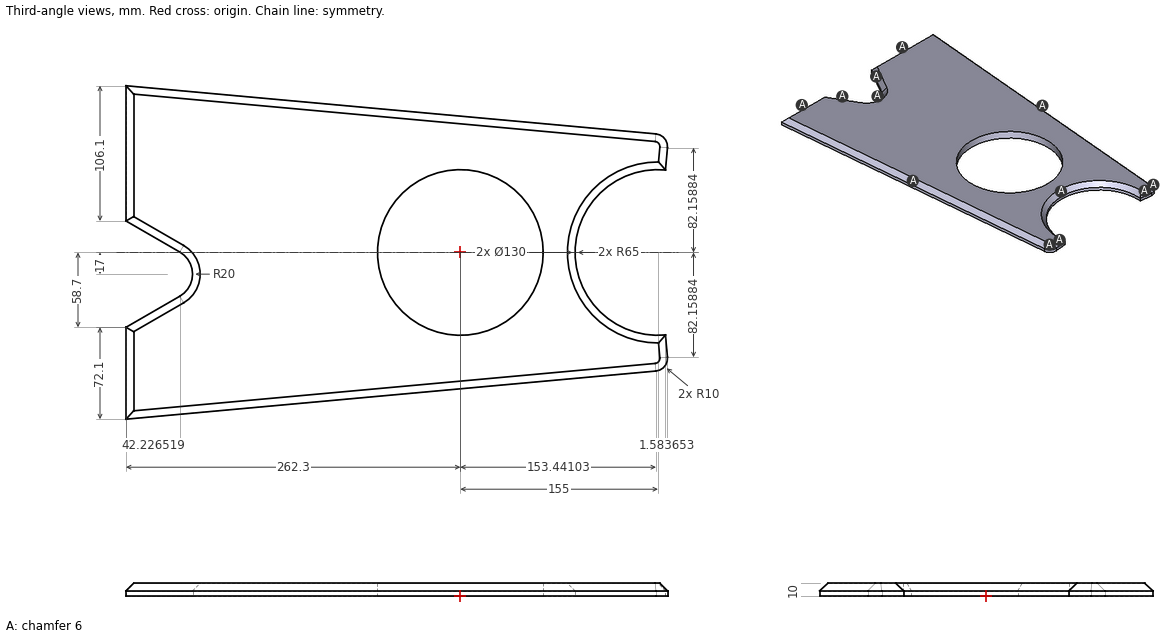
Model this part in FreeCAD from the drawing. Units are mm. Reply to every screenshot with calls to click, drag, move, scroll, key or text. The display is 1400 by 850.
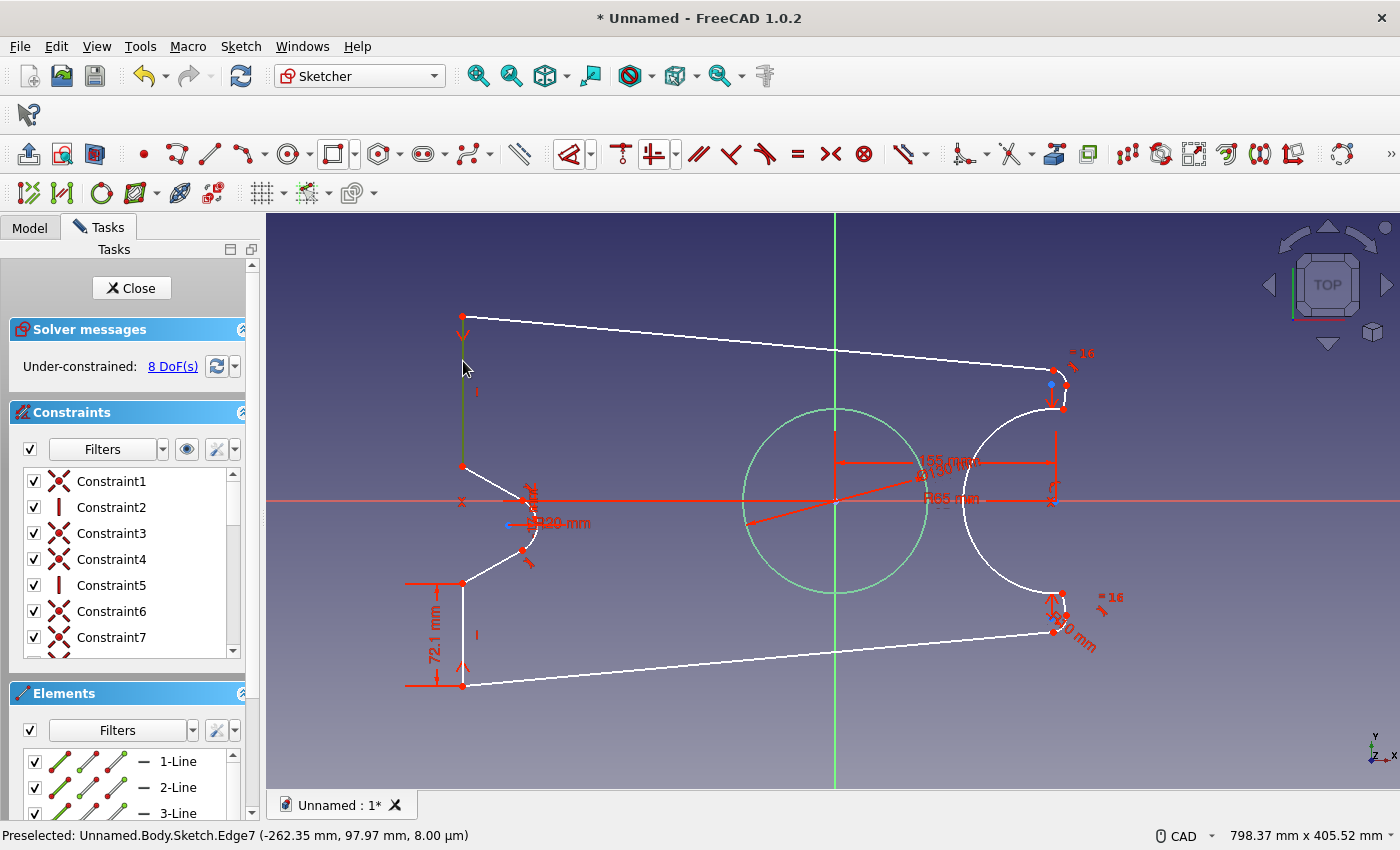
click(590, 154)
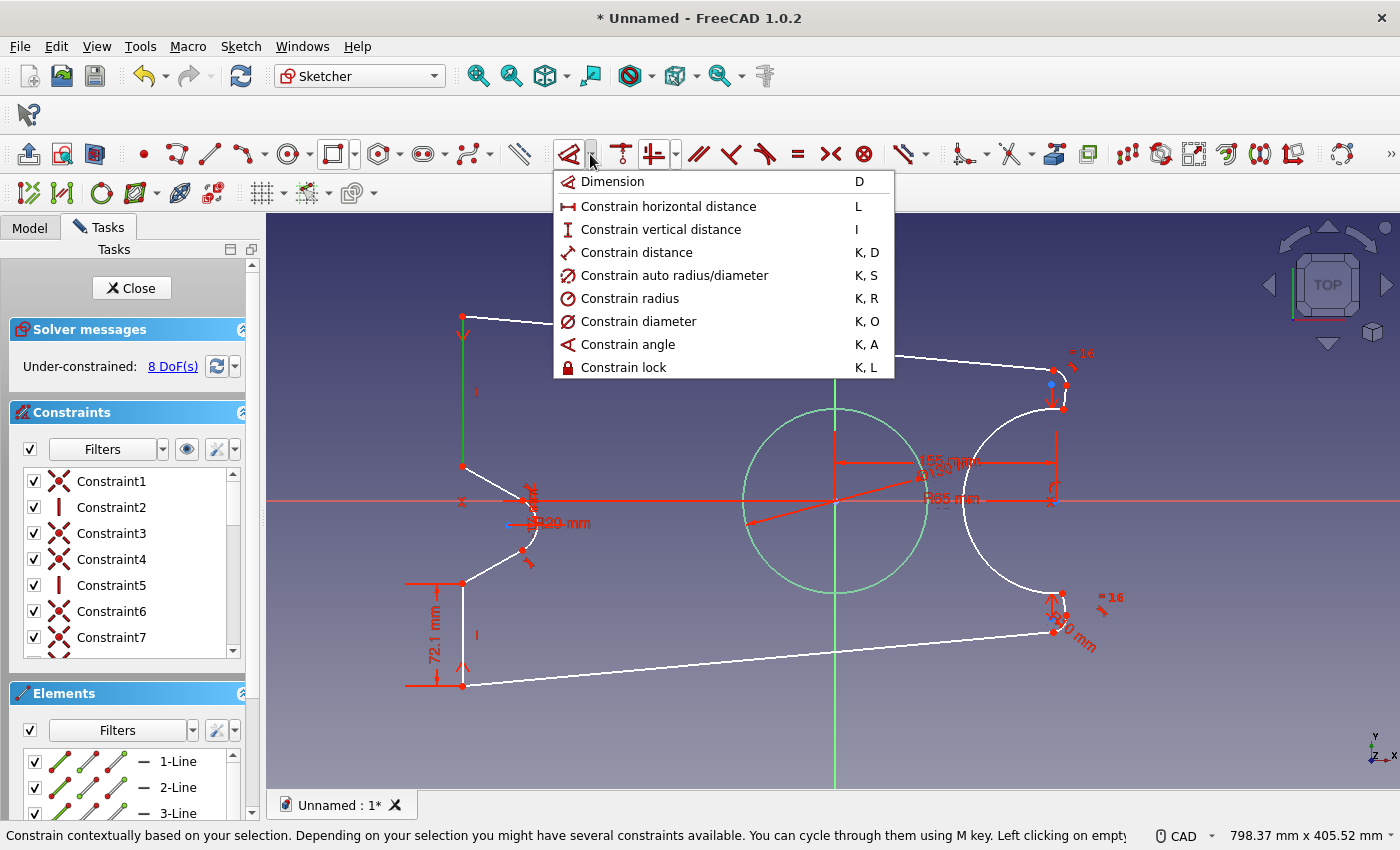
click(724, 230)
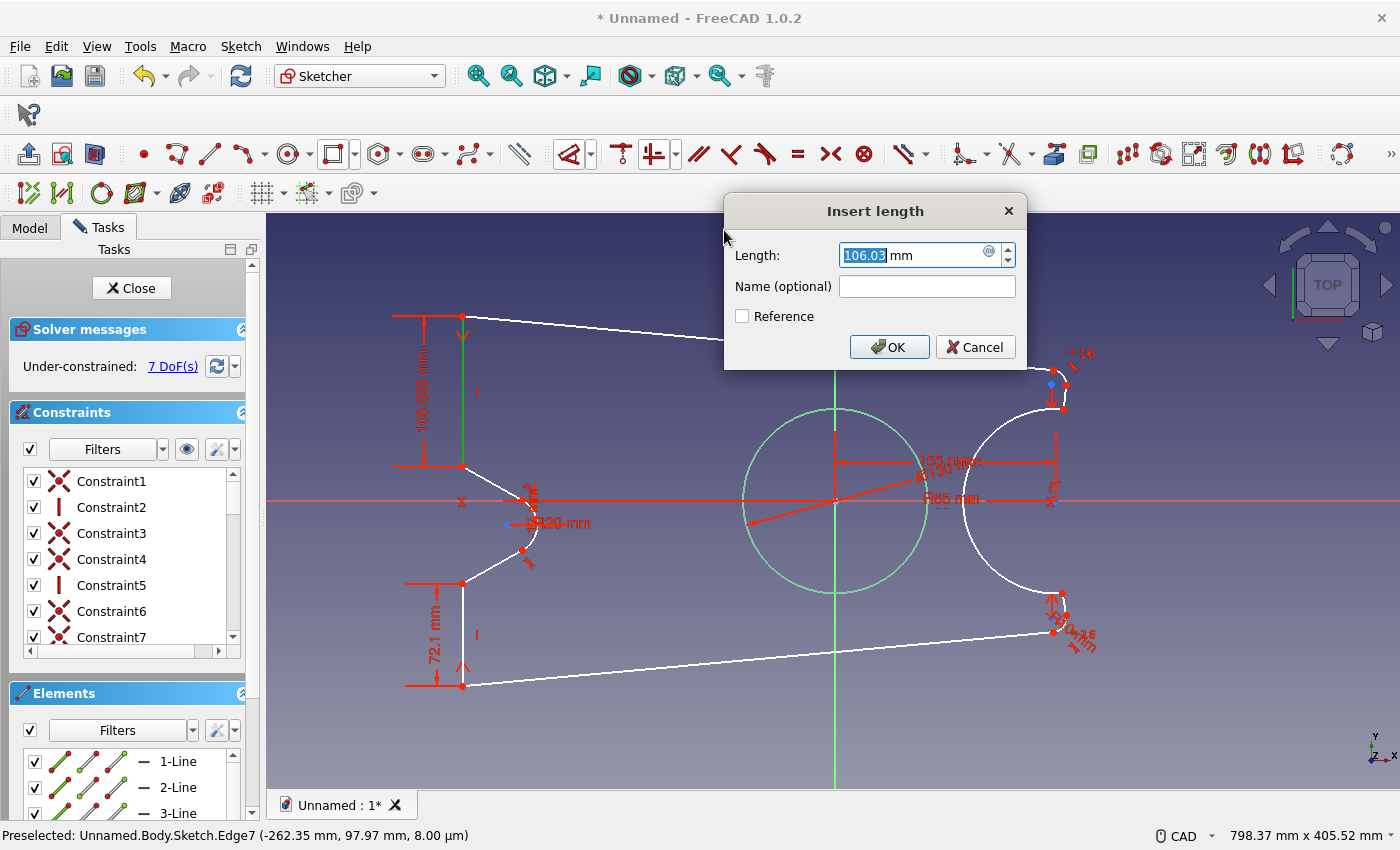
text(106.1)
key(Return)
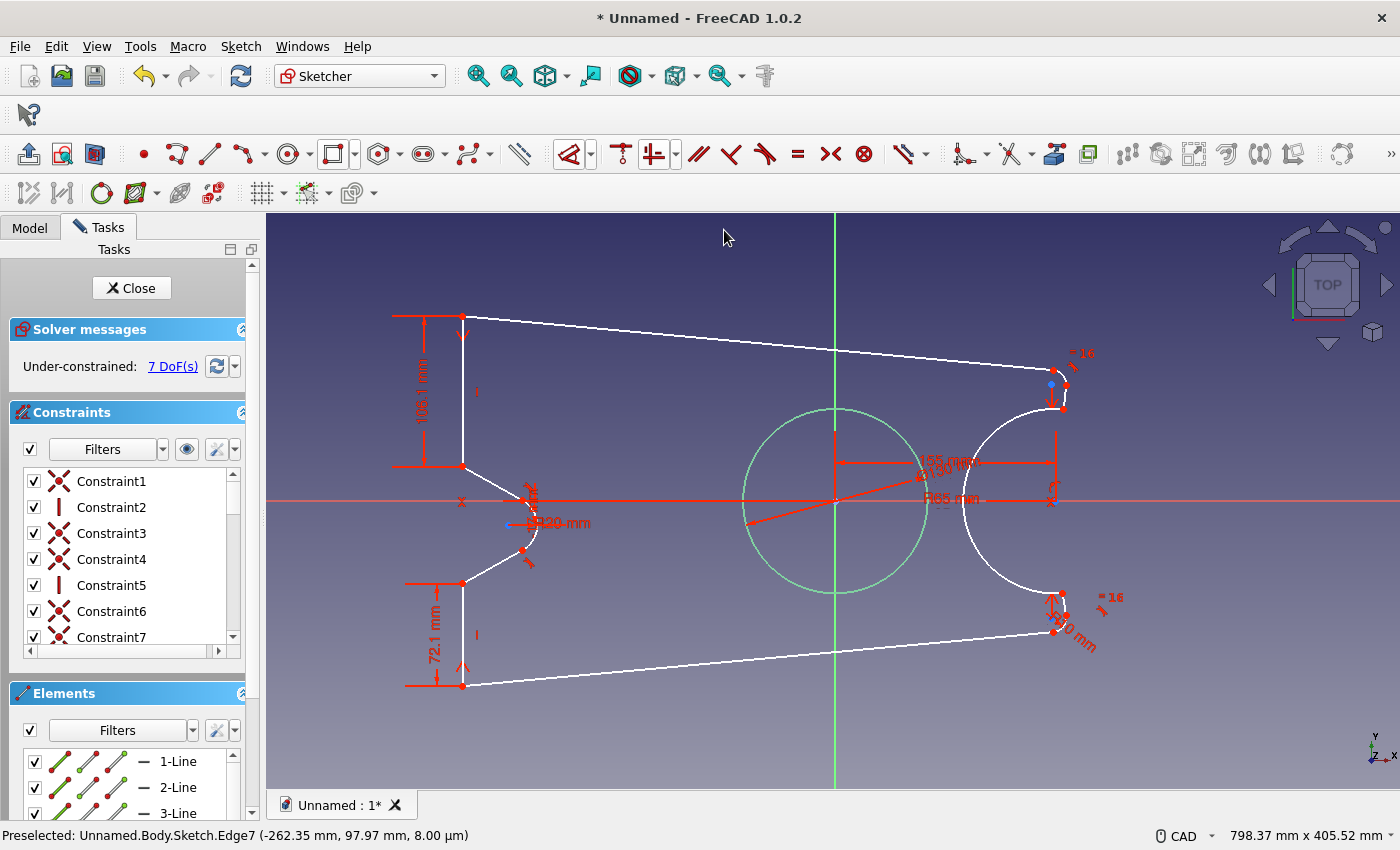
click(463, 584)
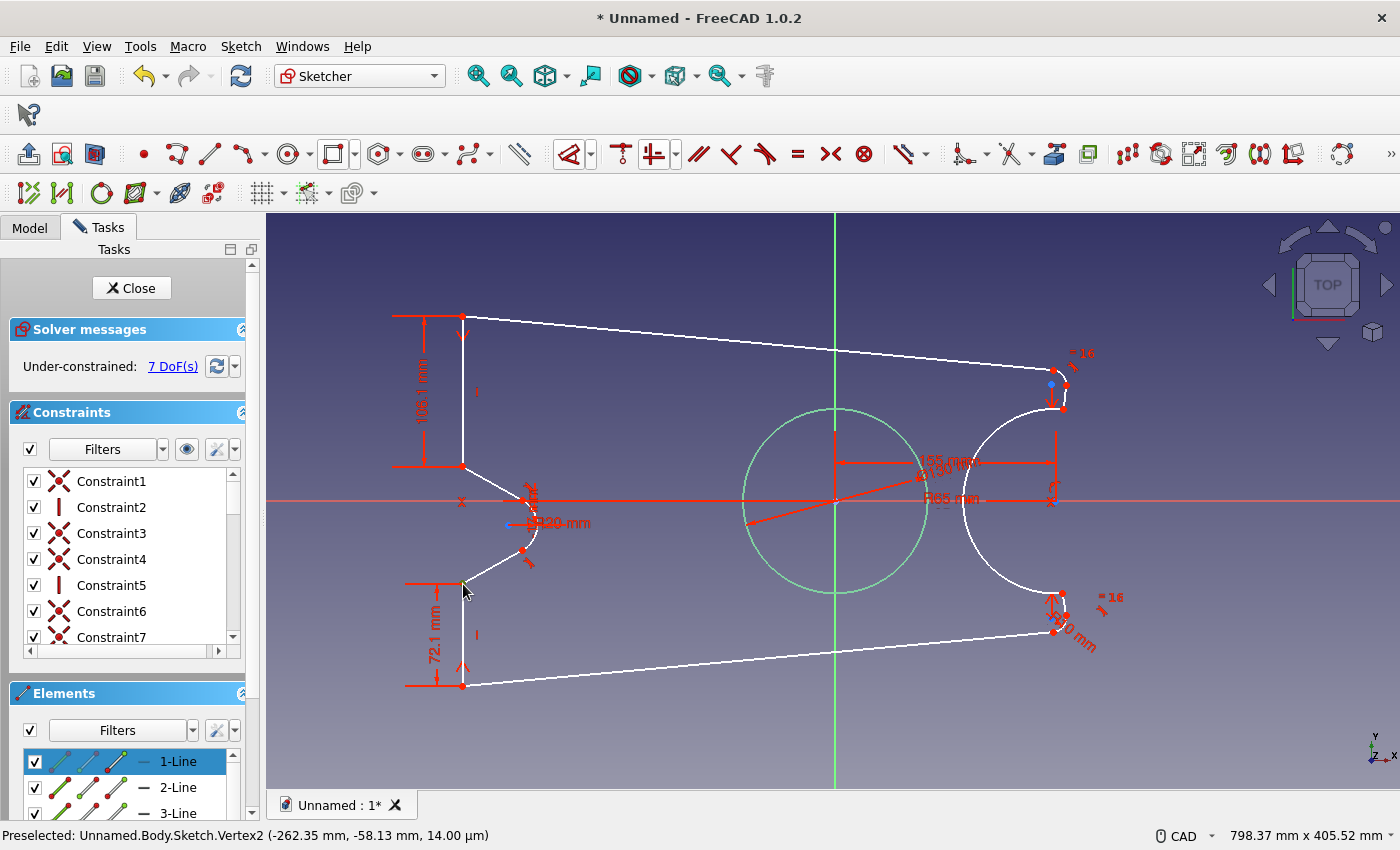
key(i)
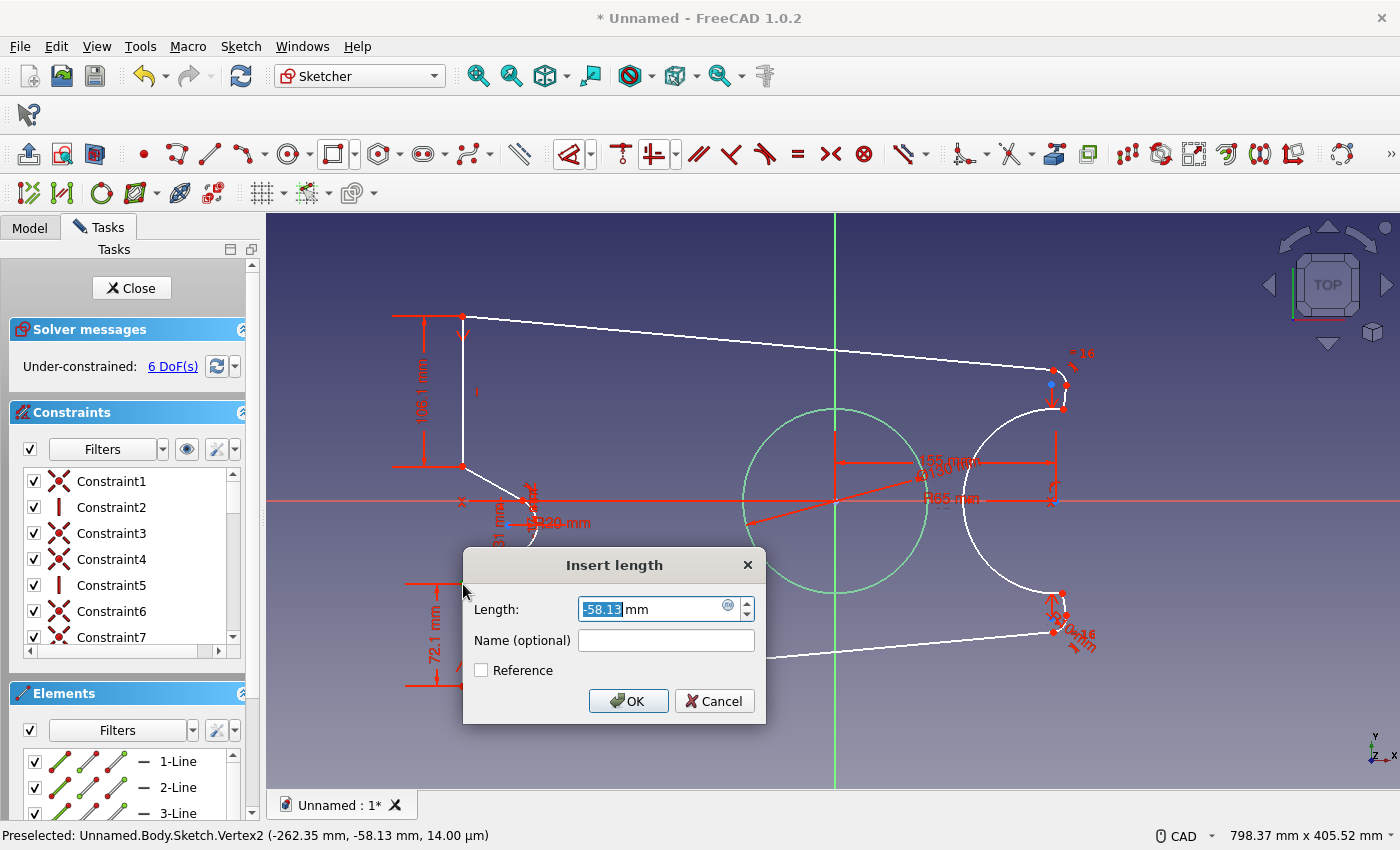
text(-58.7)
key(Return)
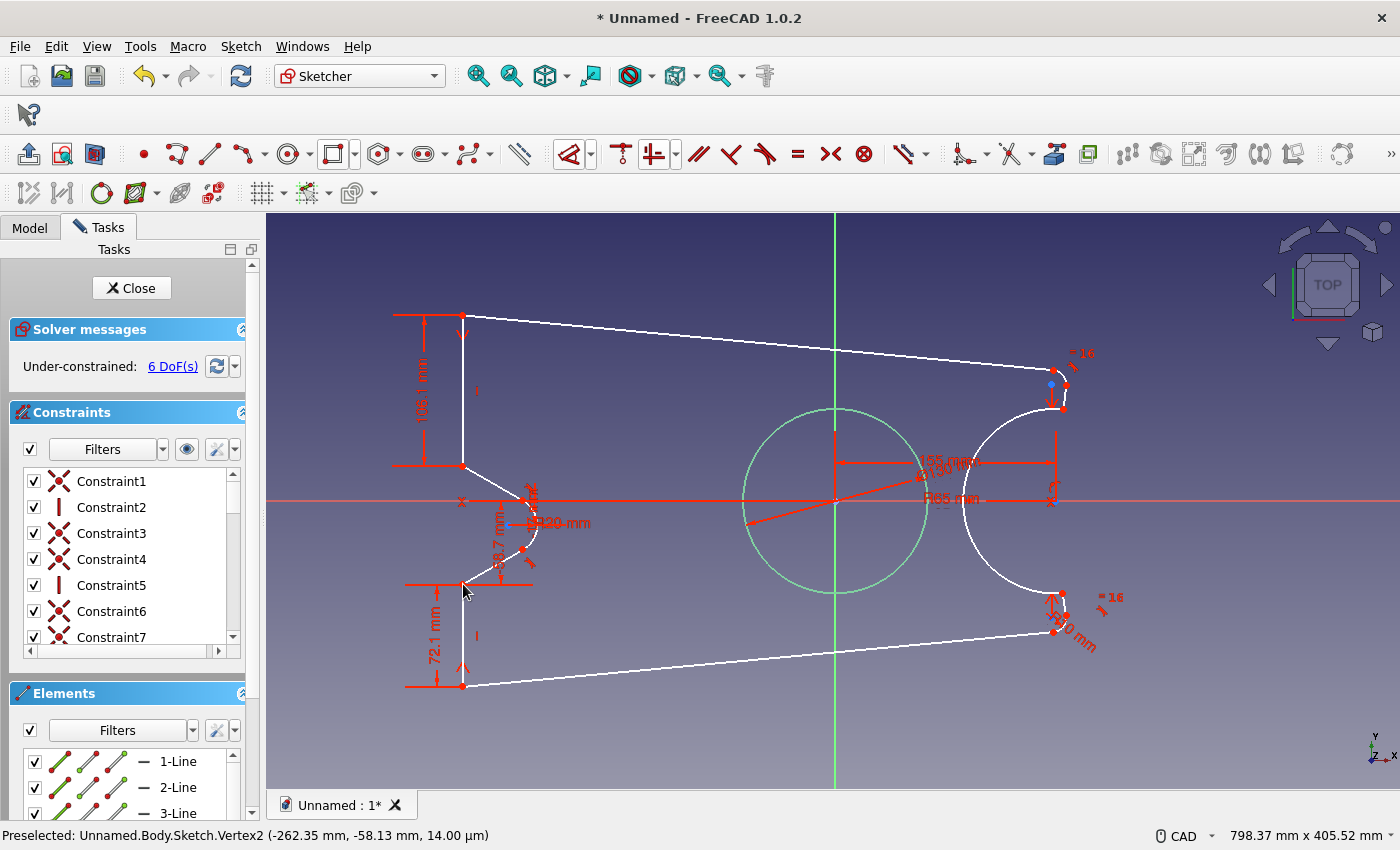
click(463, 585)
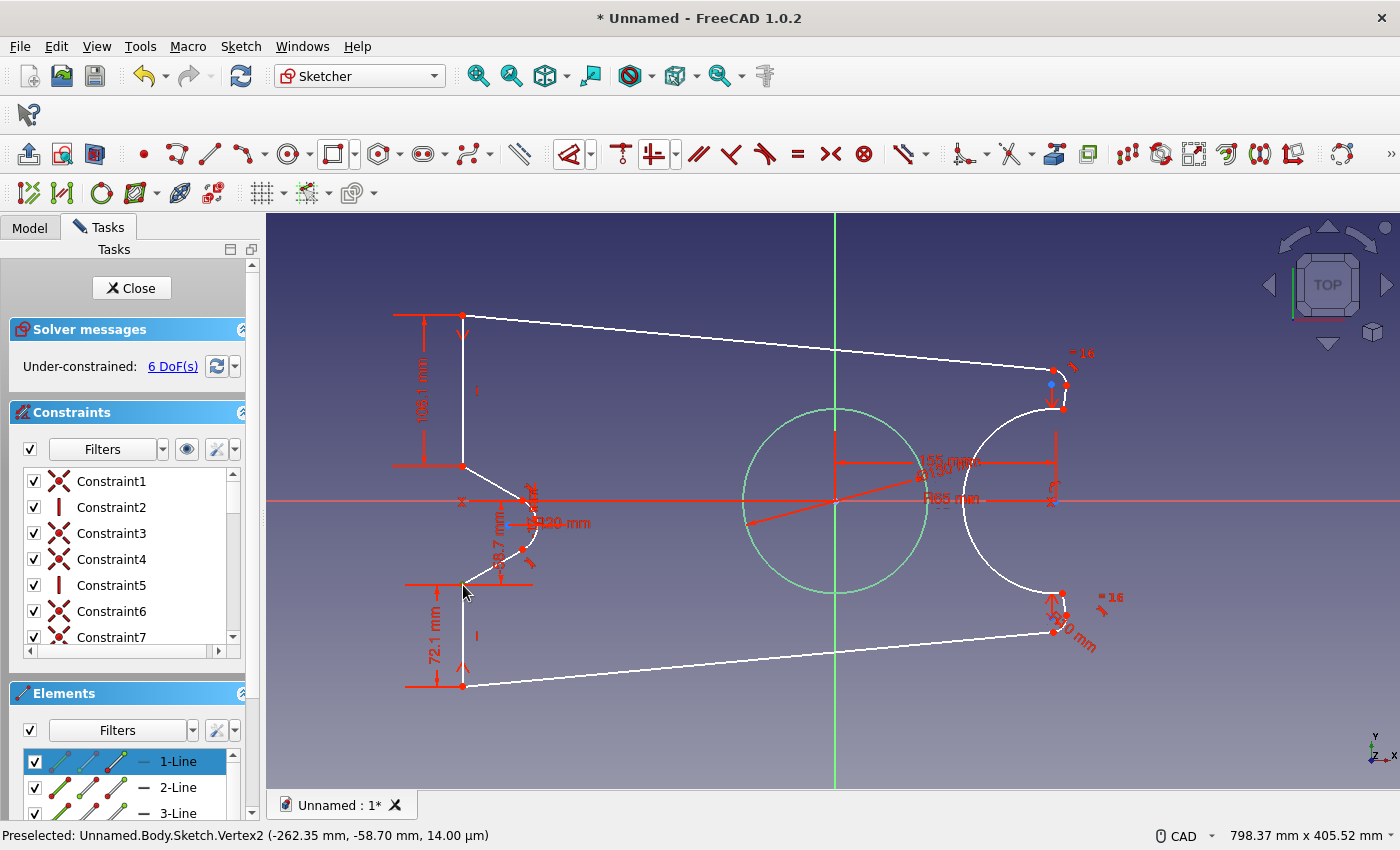
click(590, 154)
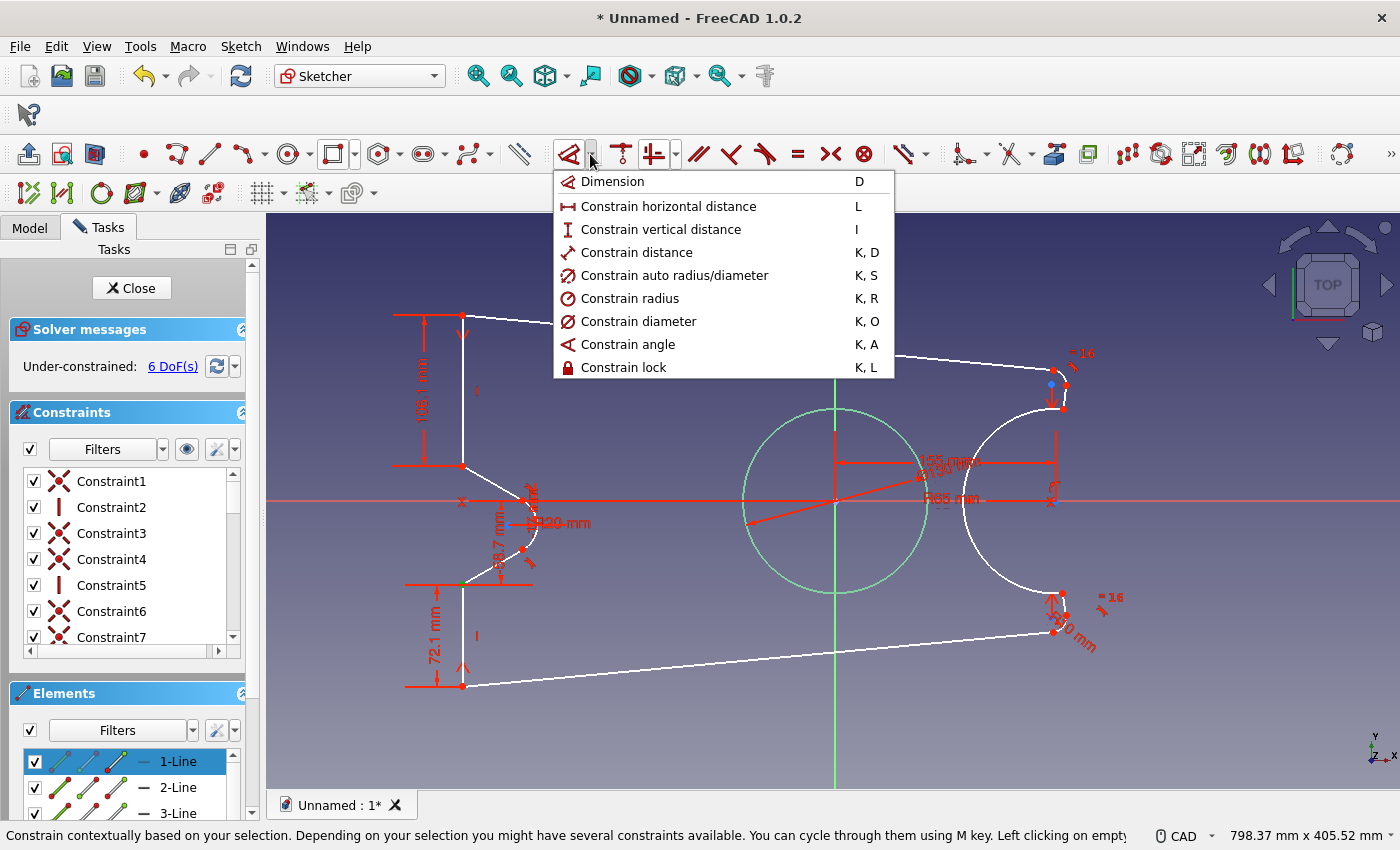
click(724, 206)